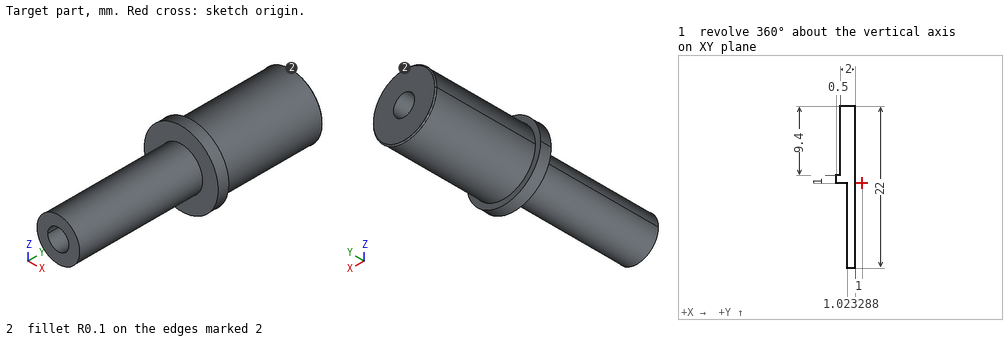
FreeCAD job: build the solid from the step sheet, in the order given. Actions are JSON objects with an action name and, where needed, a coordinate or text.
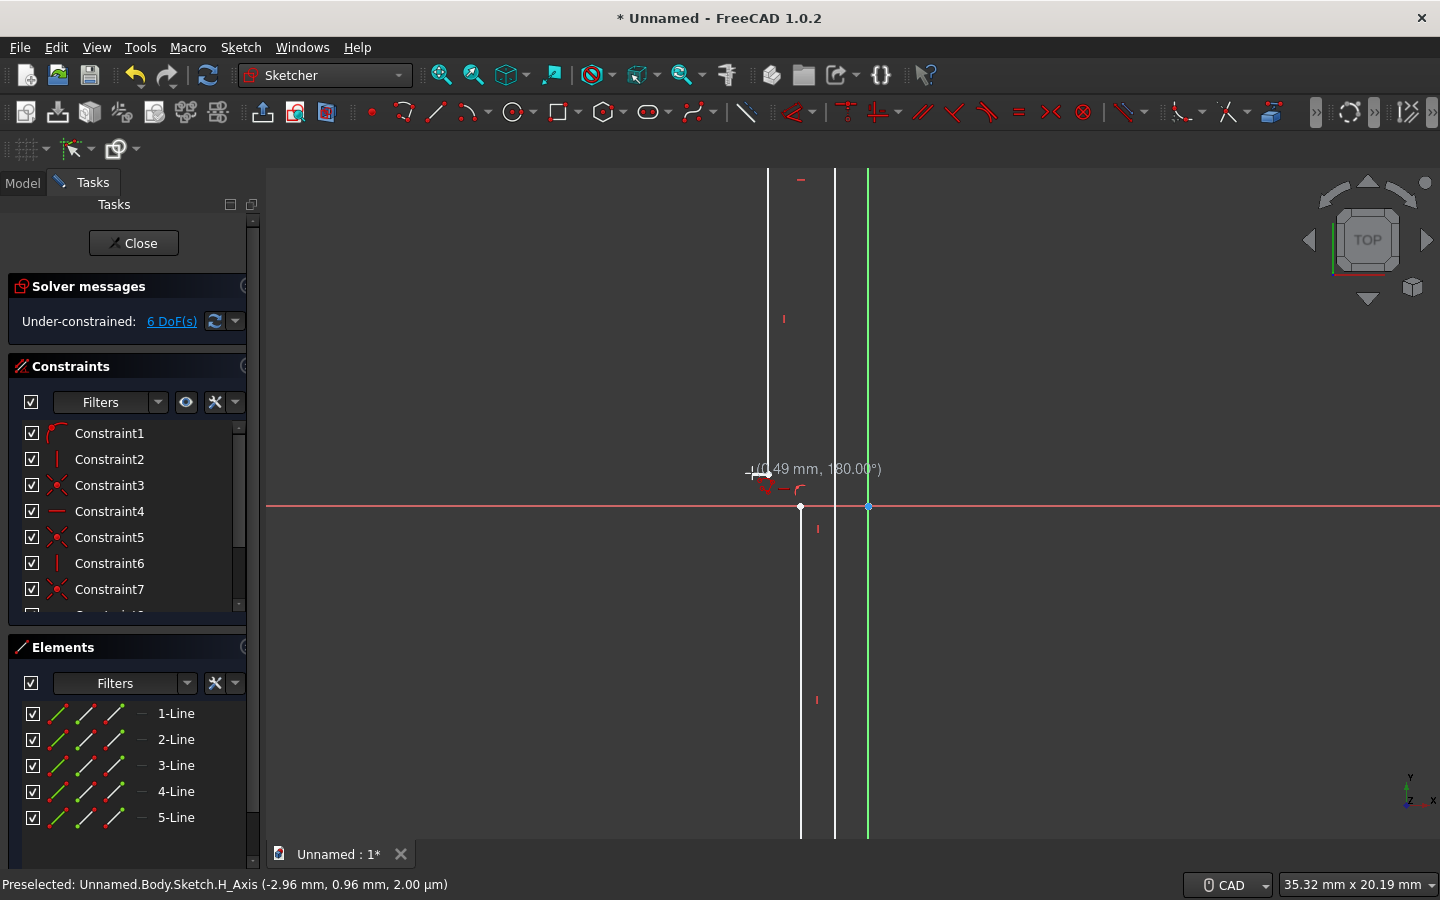
{"action": "left_click", "coordinate": [752, 473]}
{"action": "left_click", "coordinate": [752, 515]}
{"action": "left_click", "coordinate": [801, 506]}
{"action": "key", "text": "Escape"}
{"action": "key", "text": "Escape"}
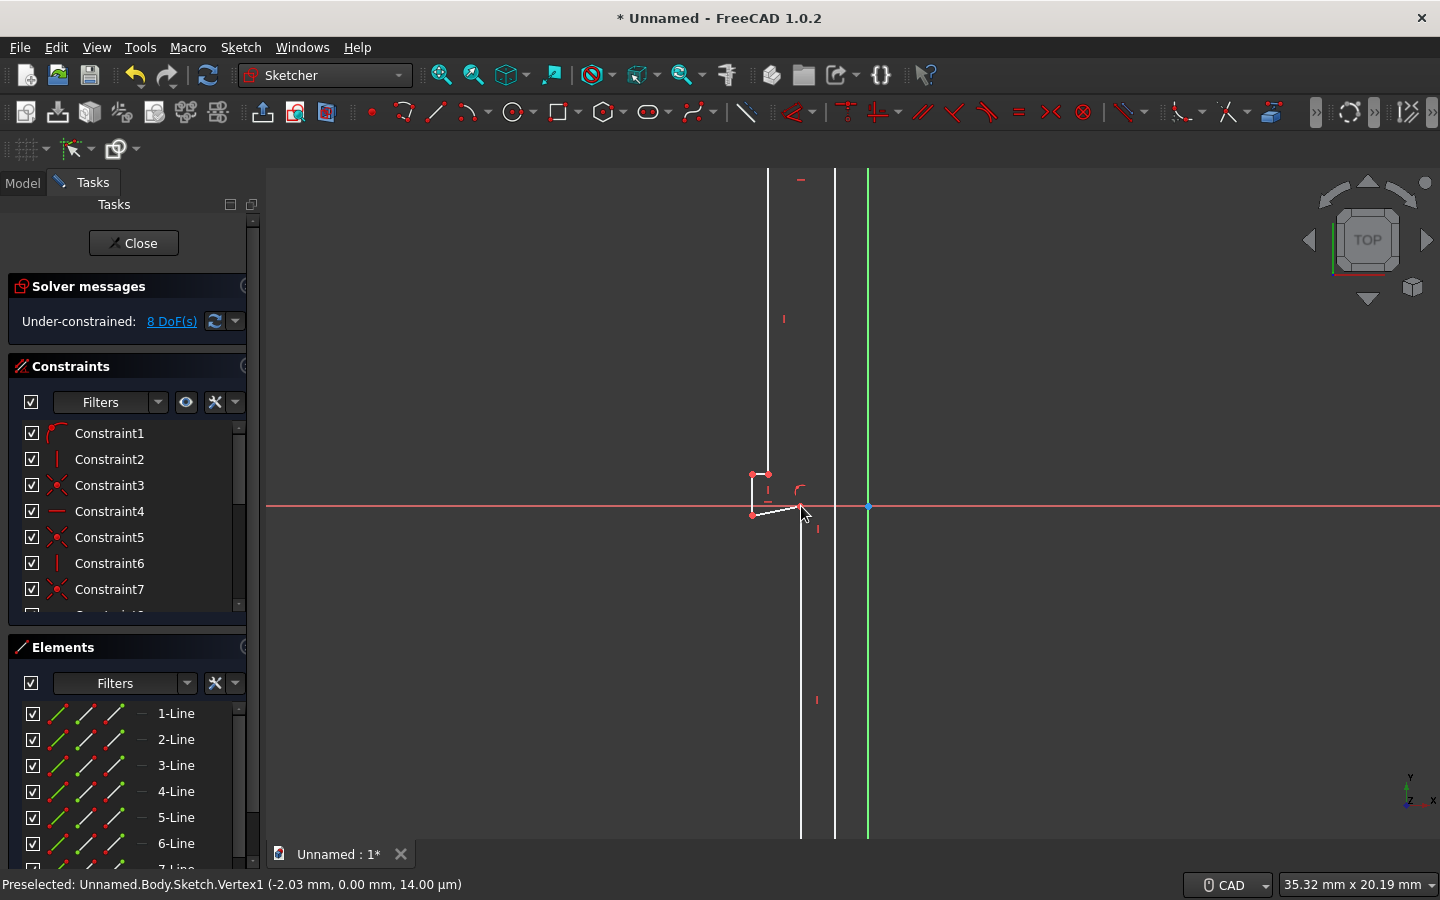
{"action": "left_click", "coordinate": [786, 509]}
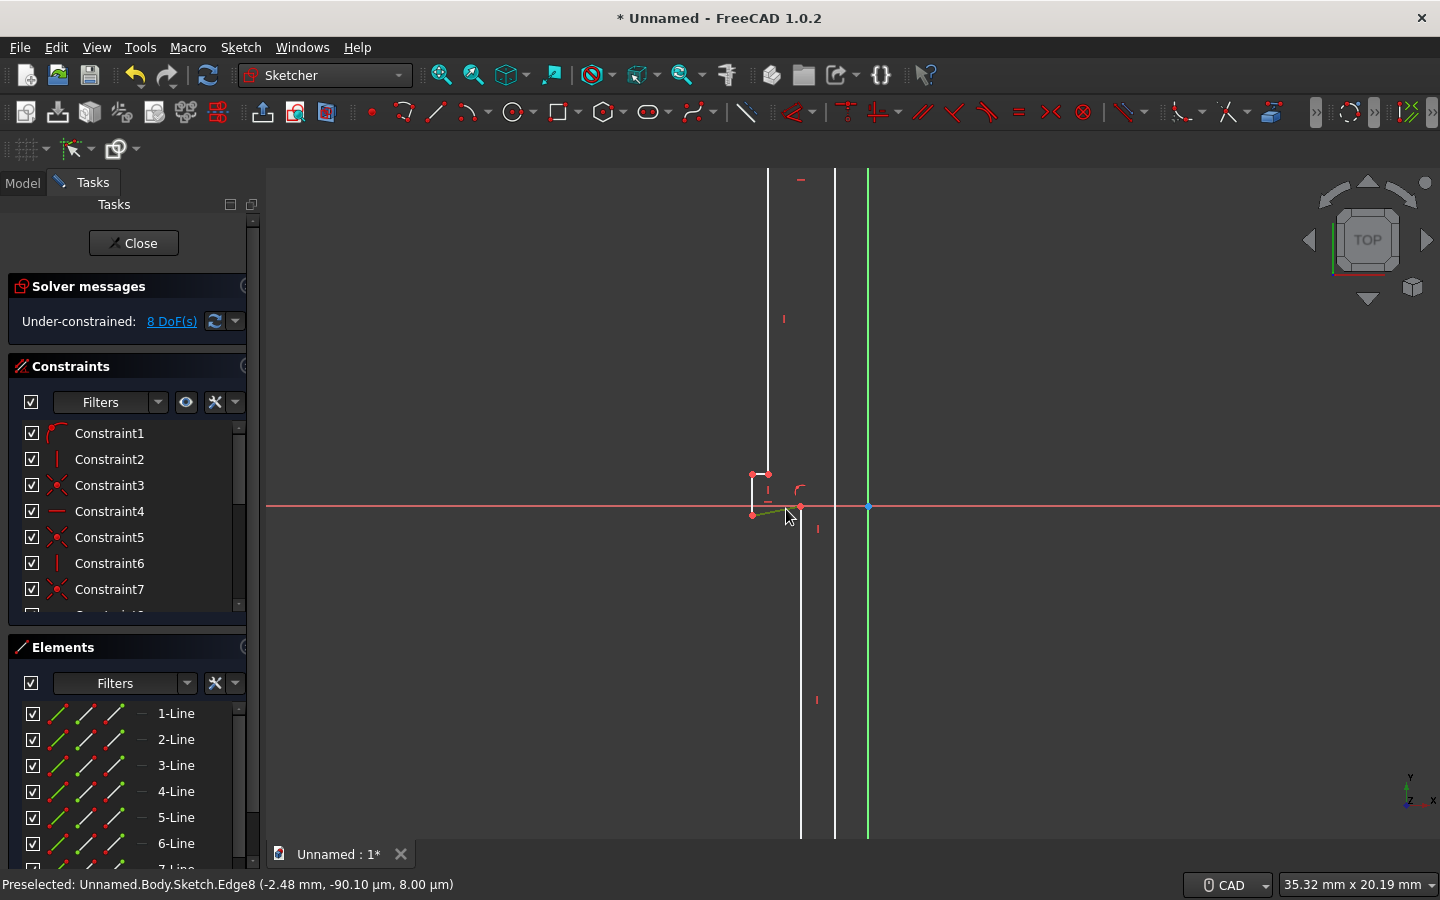
{"action": "key", "text": "h"}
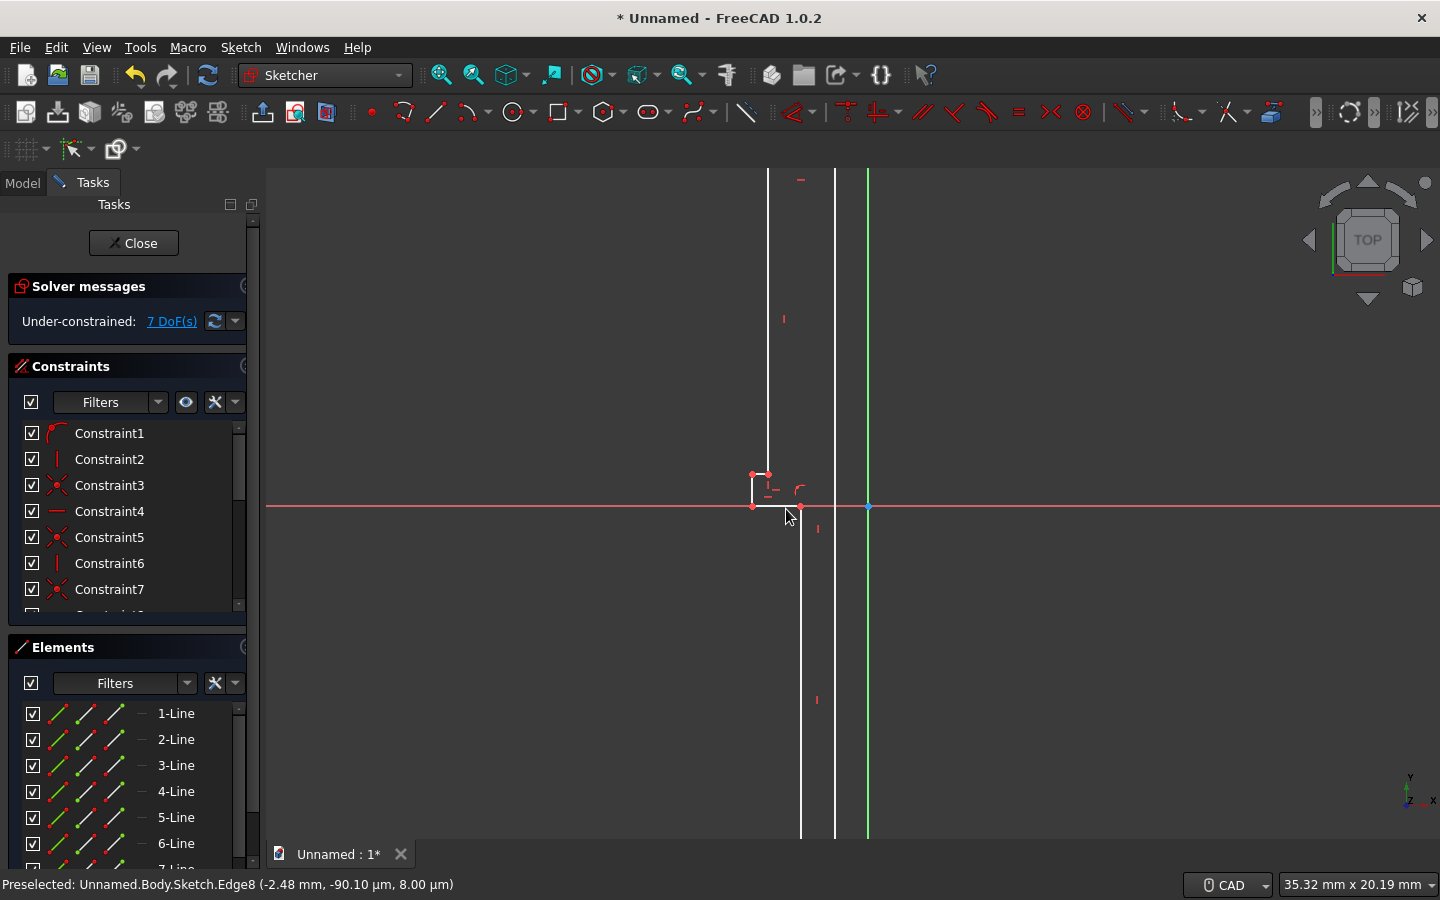
{"action": "scroll", "coordinate": [753, 476], "scroll_direction": "down", "scroll_amount": 3}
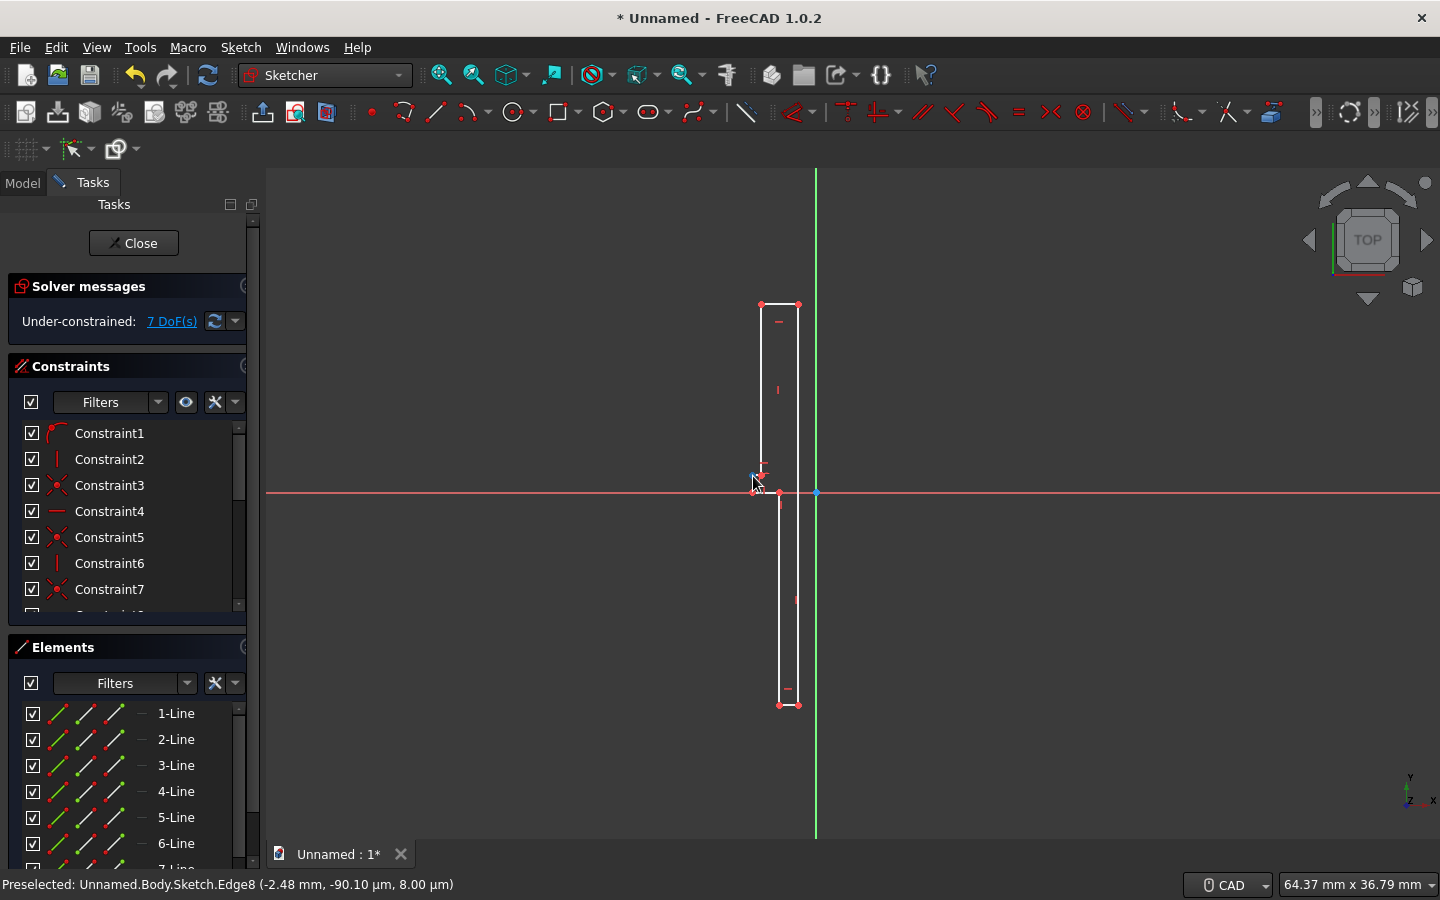
{"action": "scroll", "coordinate": [787, 304], "scroll_direction": "up", "scroll_amount": 2}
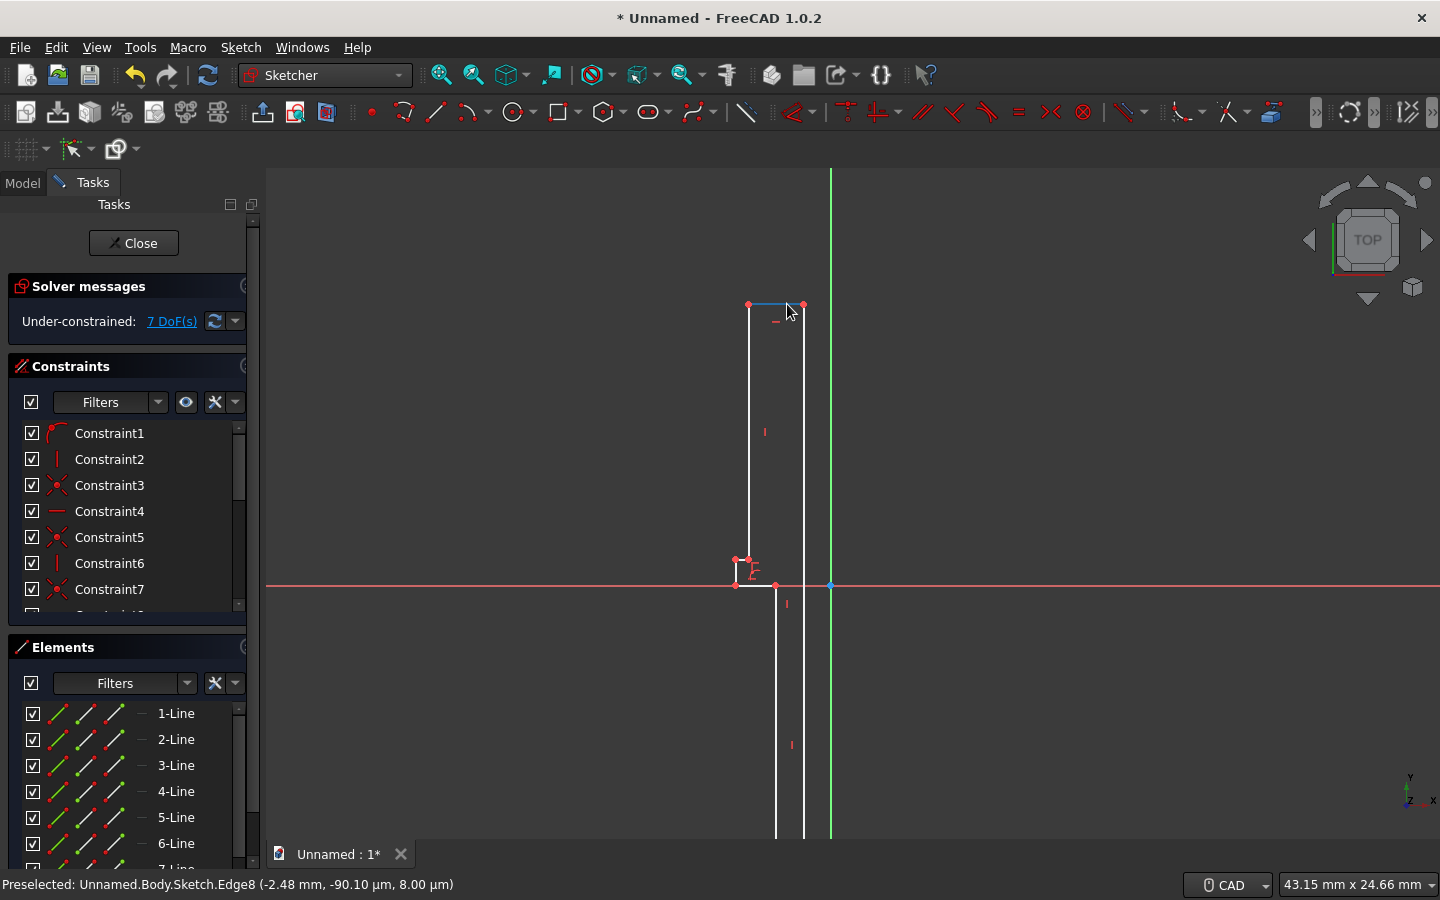
{"action": "left_click", "coordinate": [787, 304]}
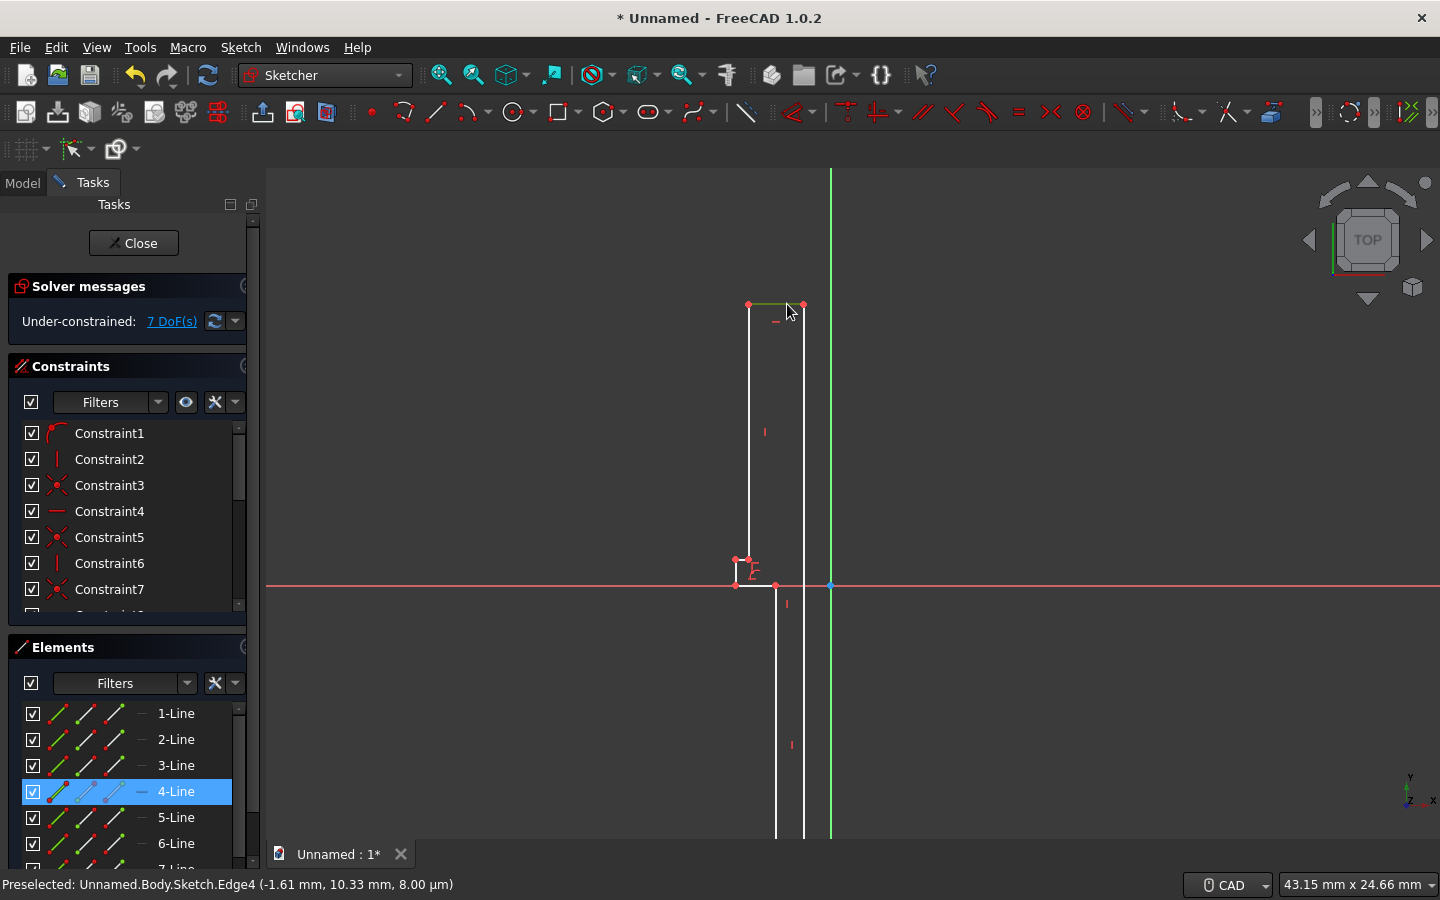
{"action": "key", "text": "l"}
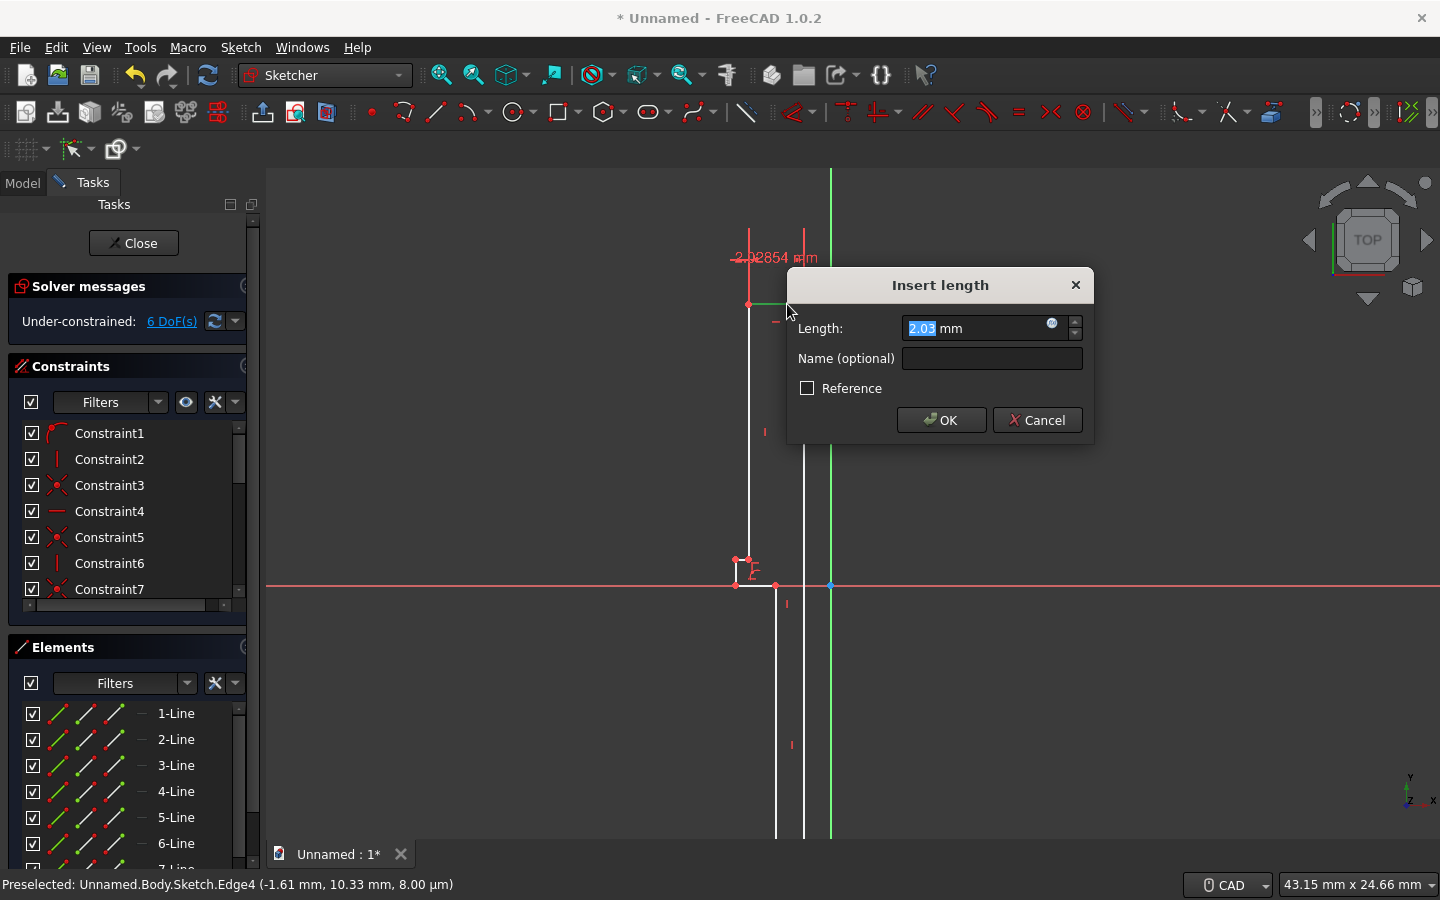
{"action": "type", "text": "2"}
{"action": "key", "text": "Return"}